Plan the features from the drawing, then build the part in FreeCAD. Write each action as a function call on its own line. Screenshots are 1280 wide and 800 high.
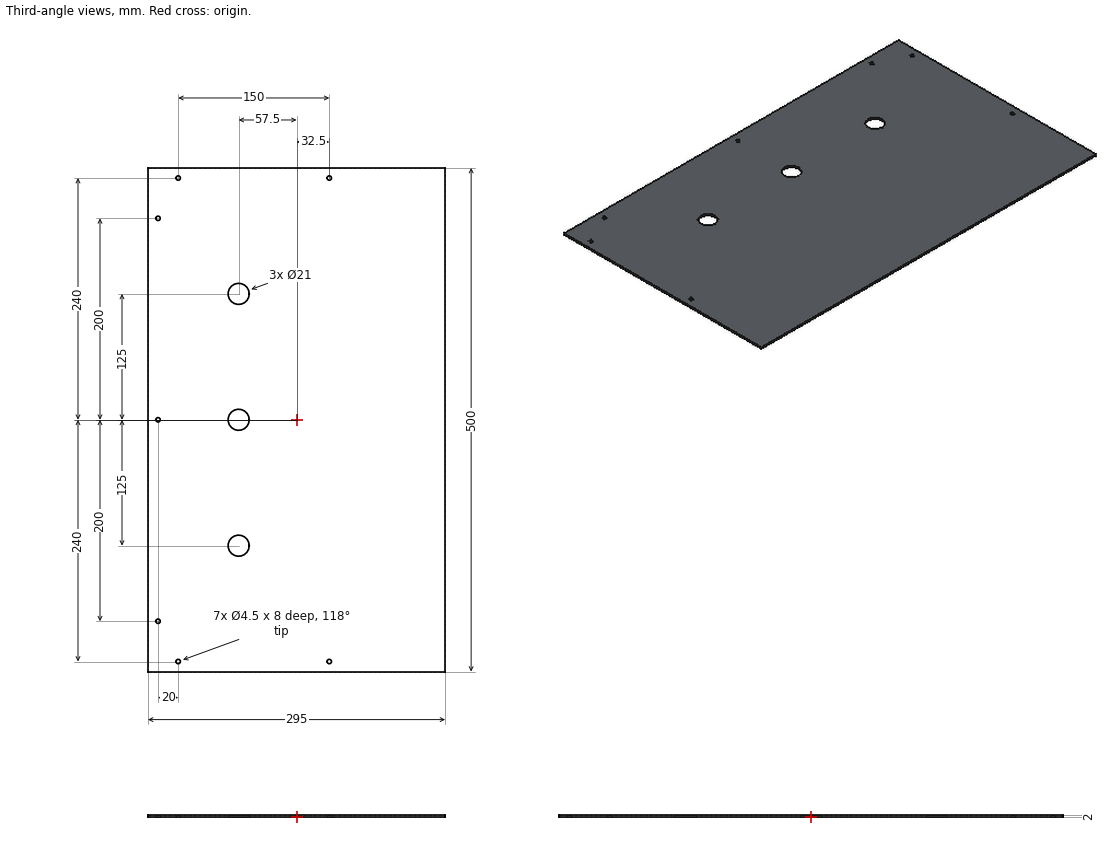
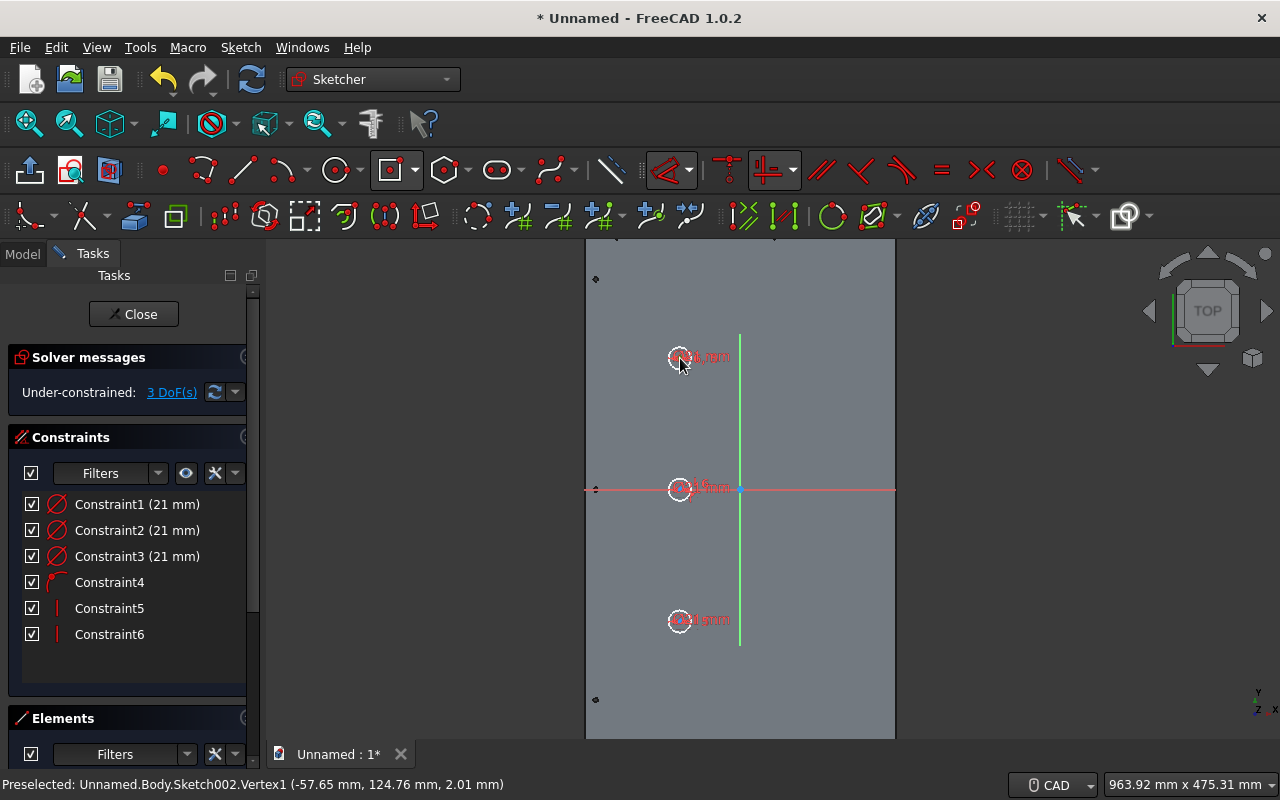
key(i)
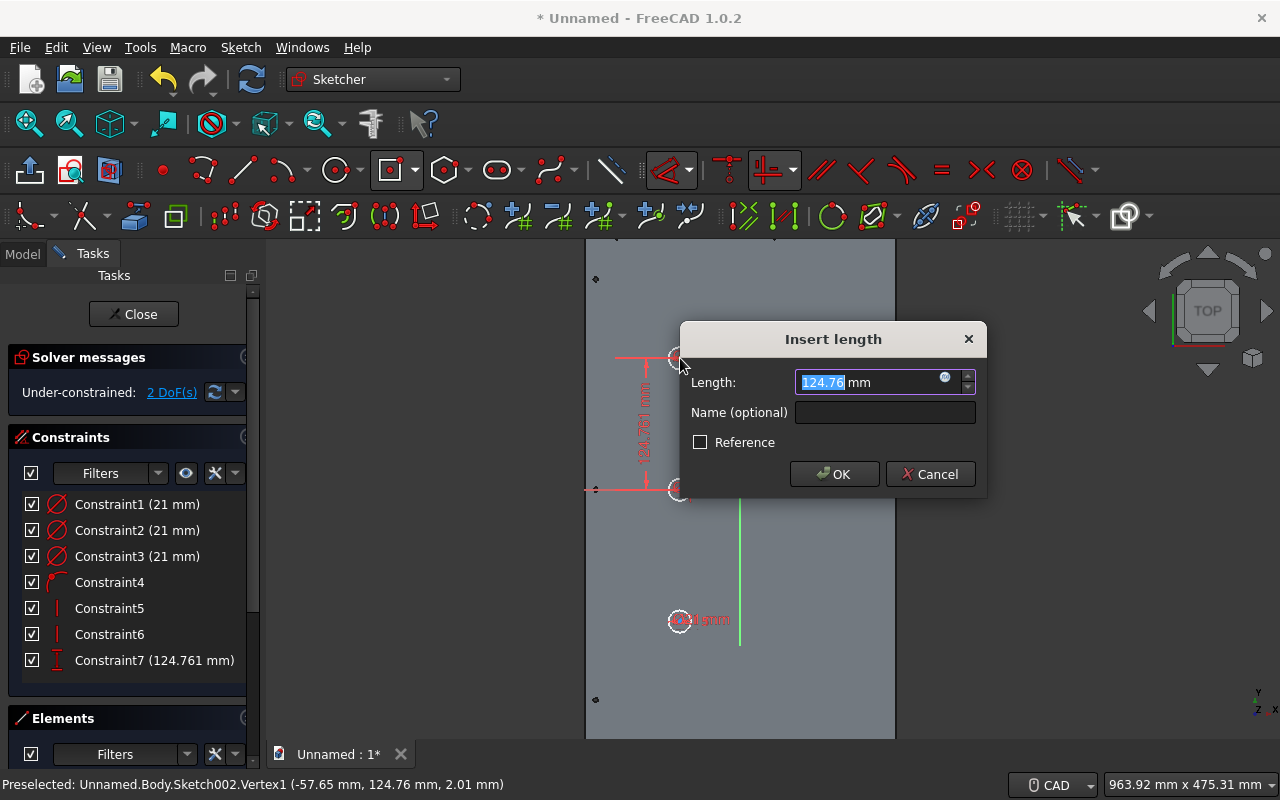
text(125)
key(Return)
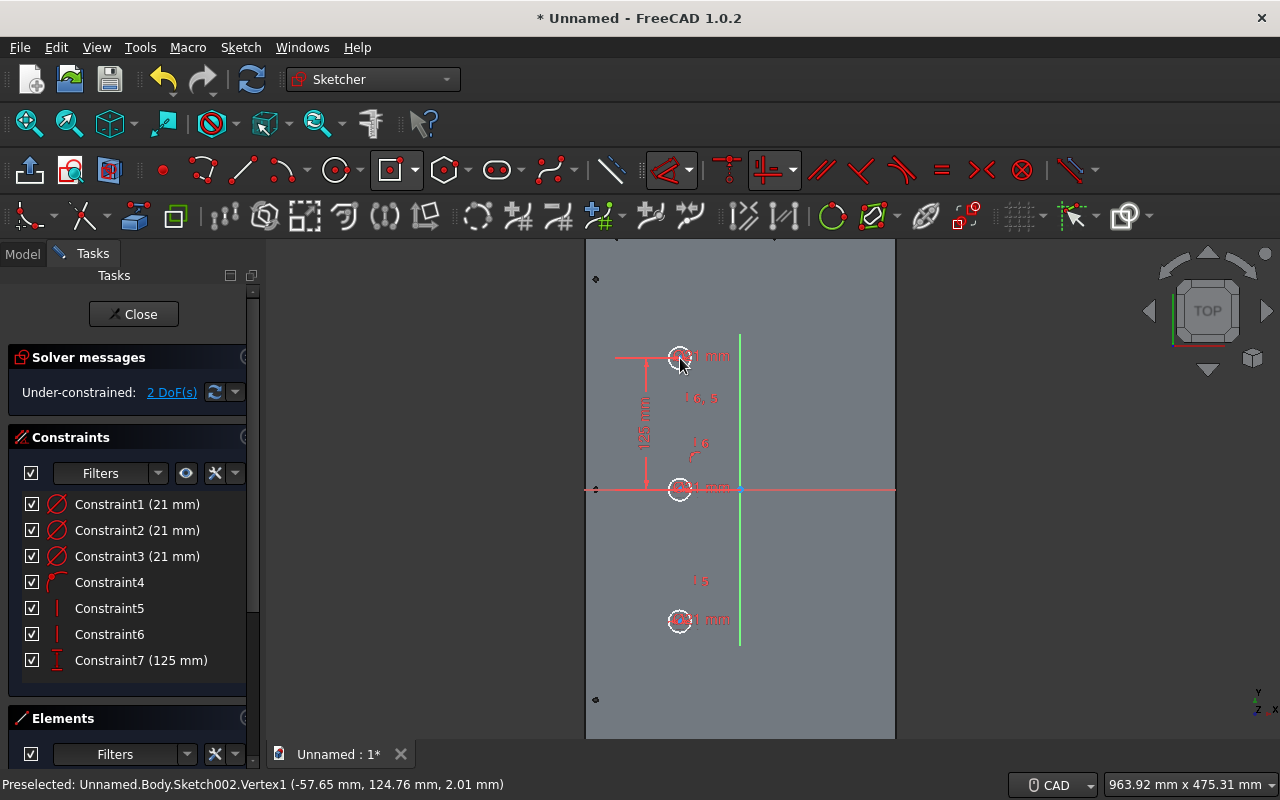
click(680, 622)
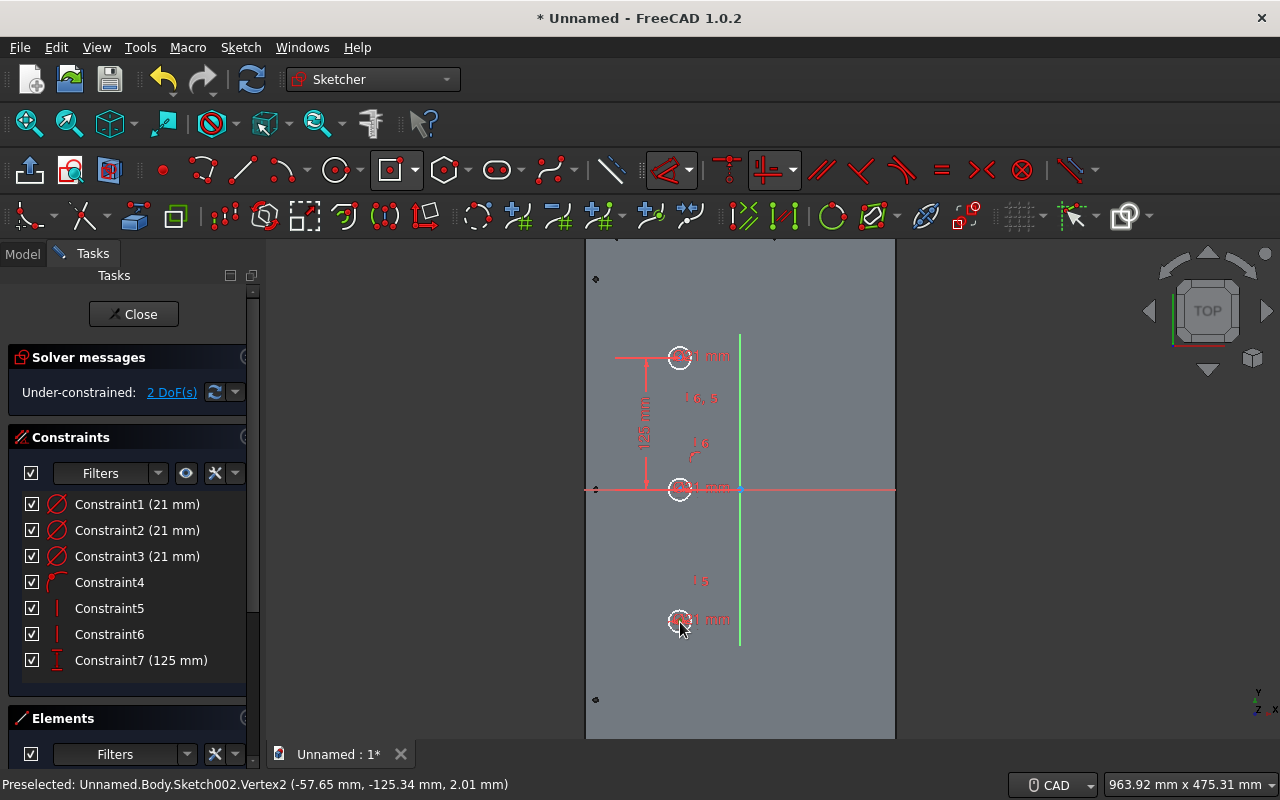
key(i)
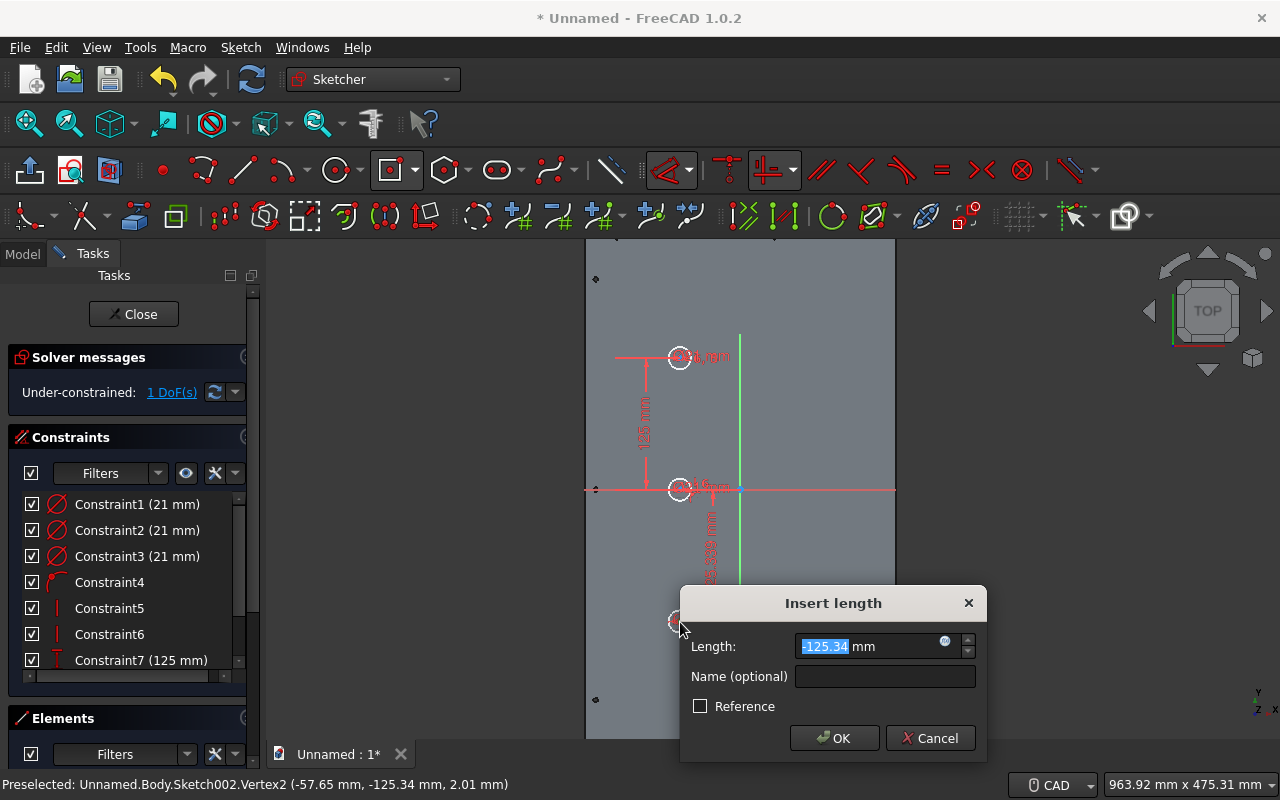
text(-125)
key(Return)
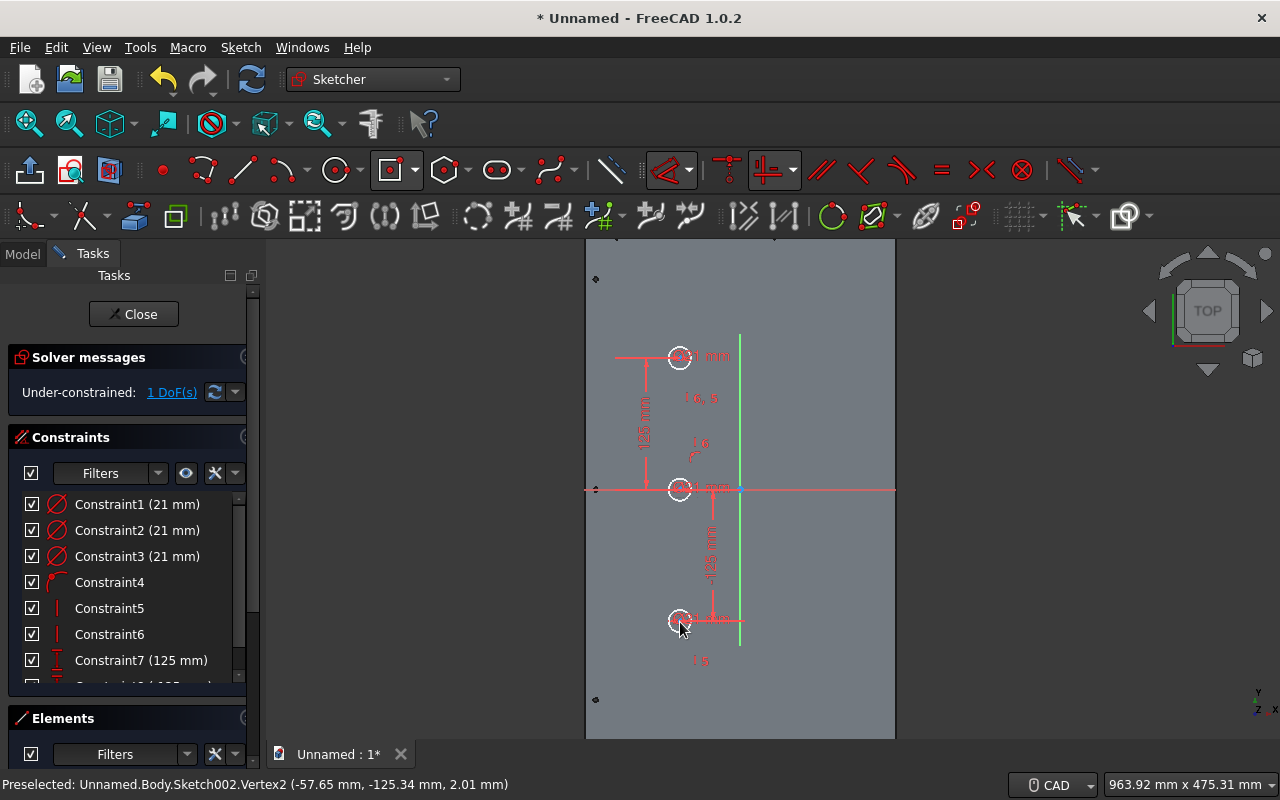
click(680, 358)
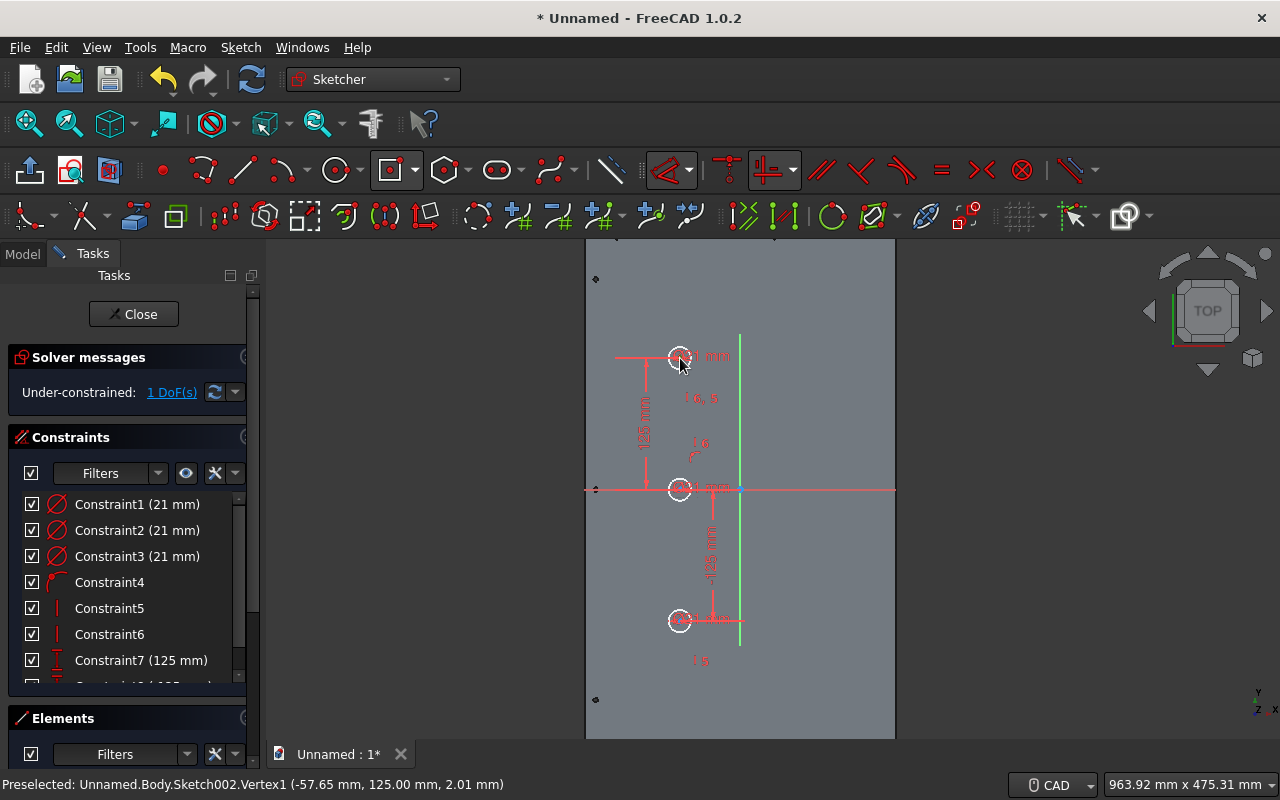
click(692, 170)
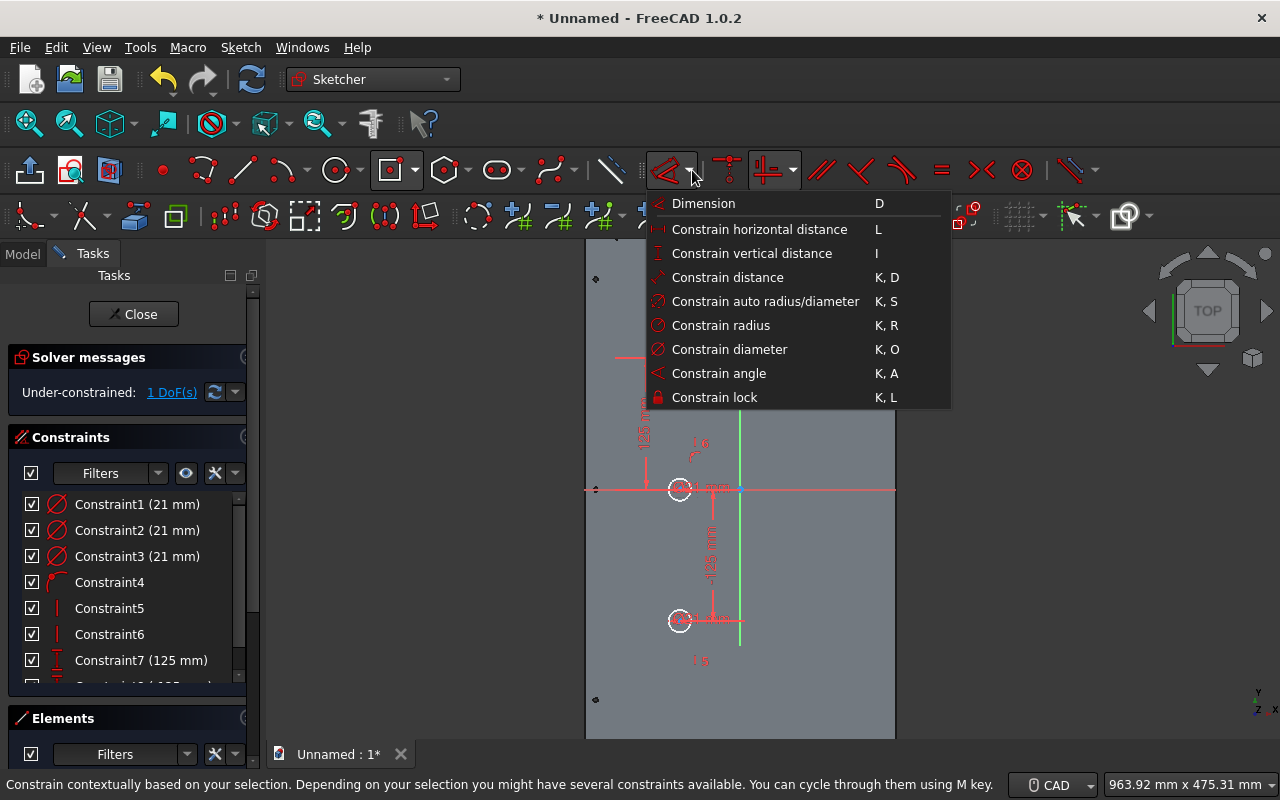
click(799, 229)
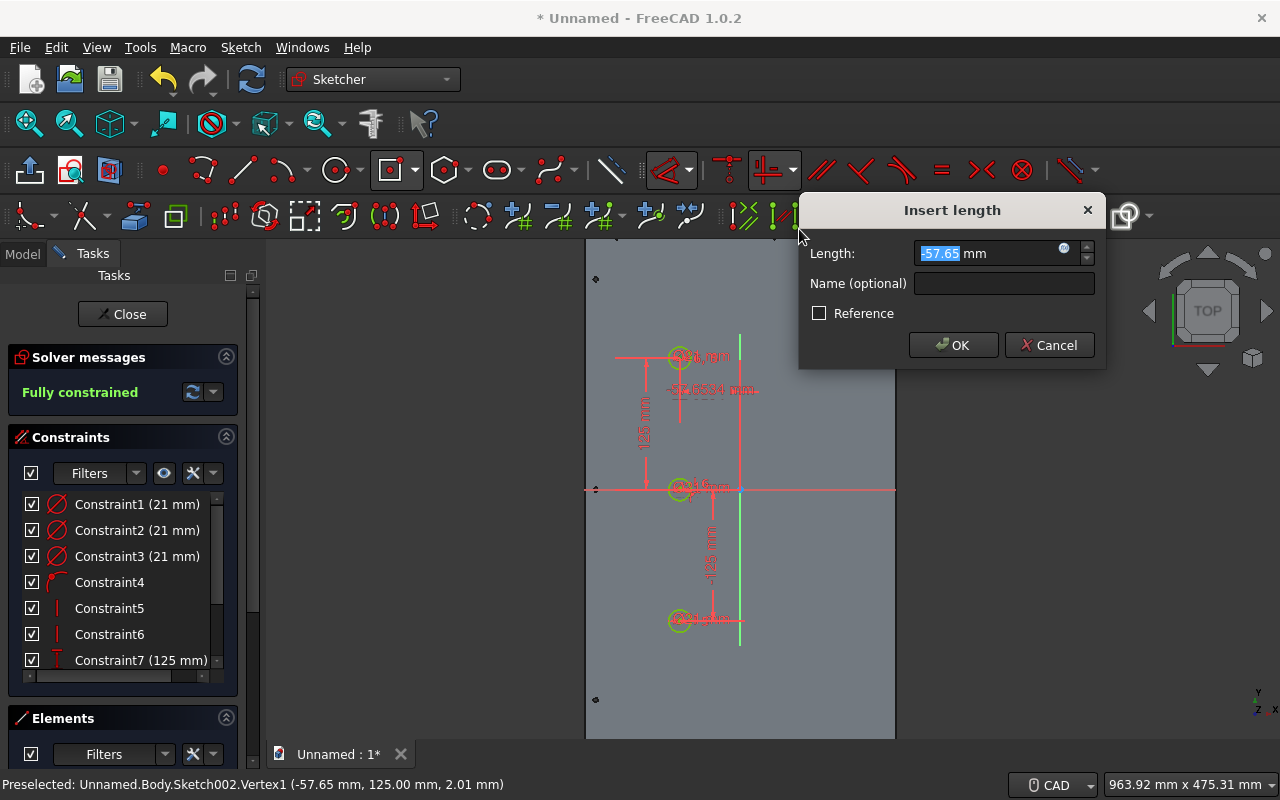
text(-57.5)
key(Return)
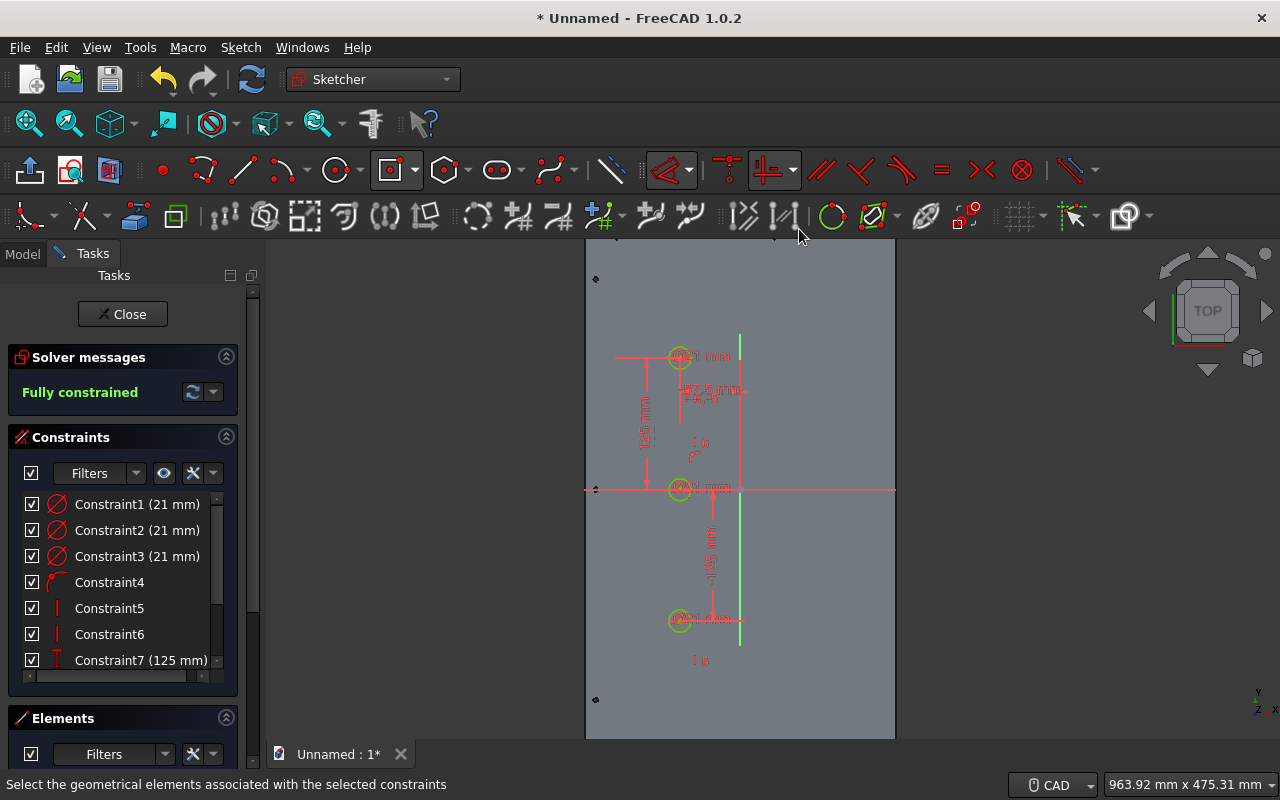
click(123, 314)